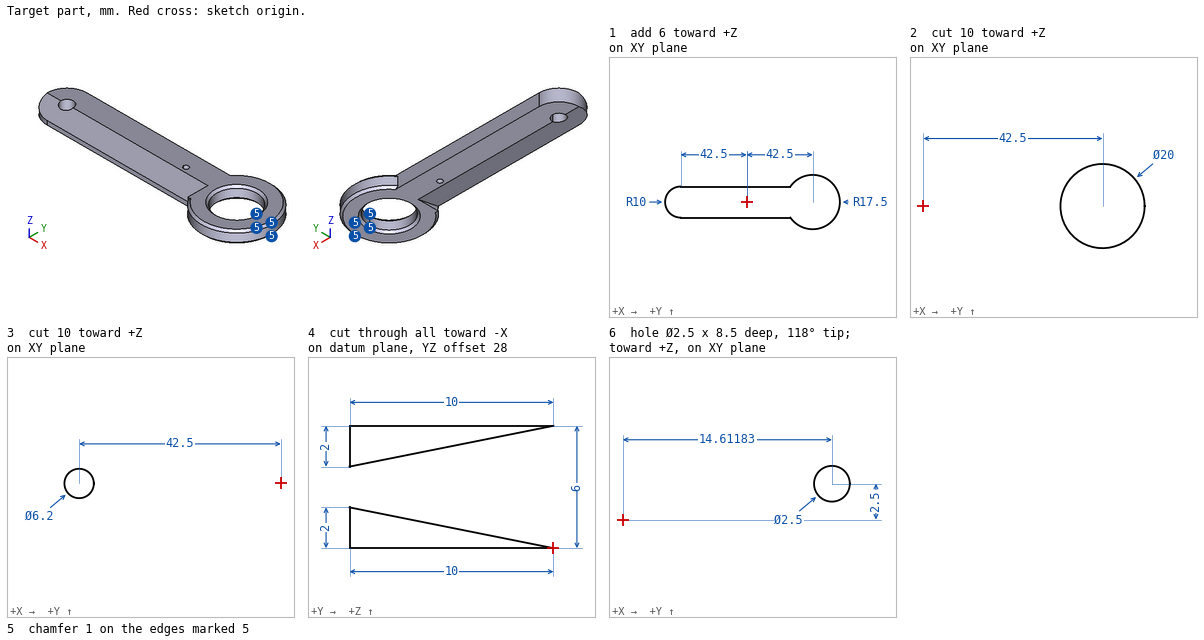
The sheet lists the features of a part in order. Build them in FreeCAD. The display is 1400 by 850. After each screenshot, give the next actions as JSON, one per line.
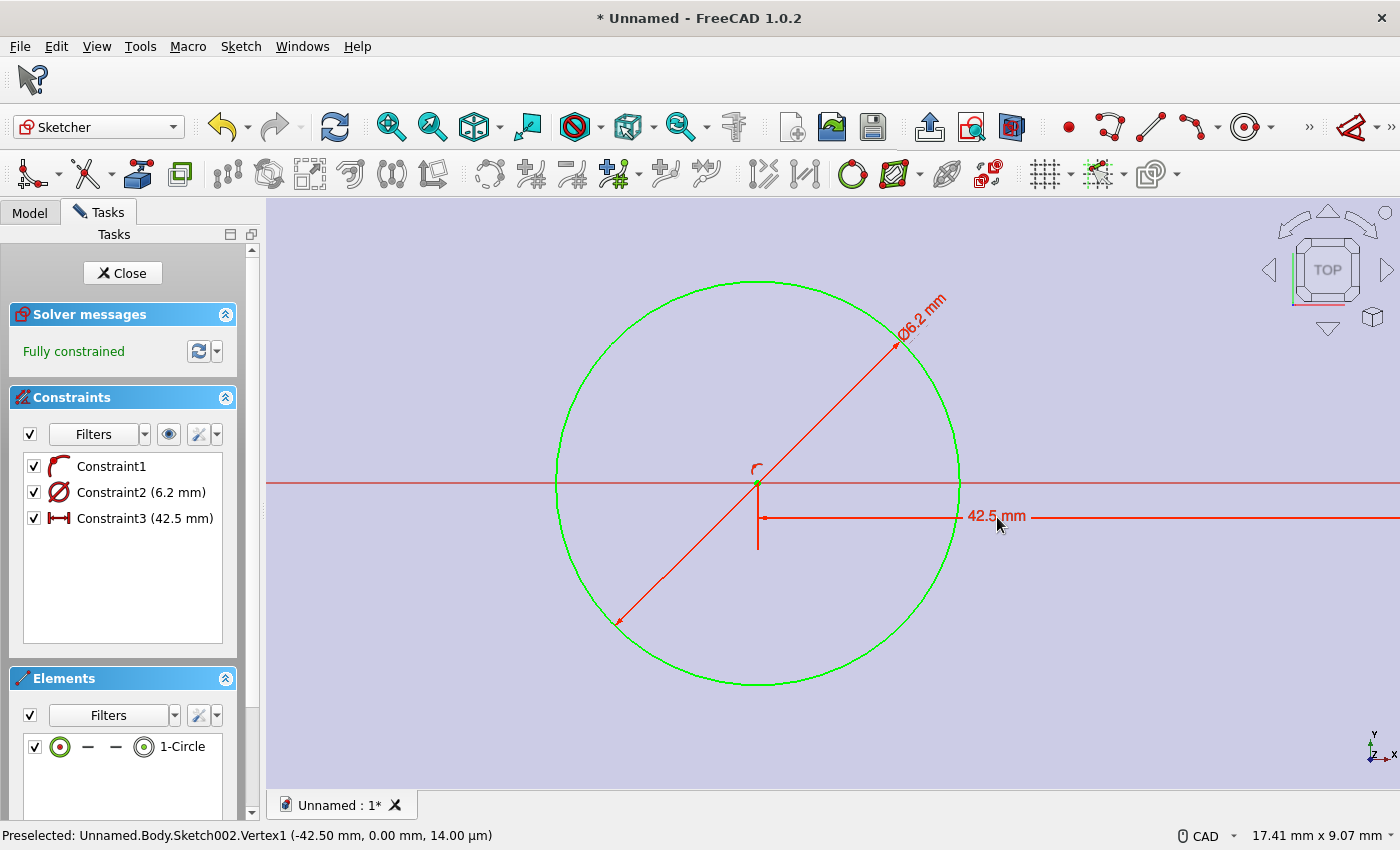
{"action": "left_click", "coordinate": [123, 273]}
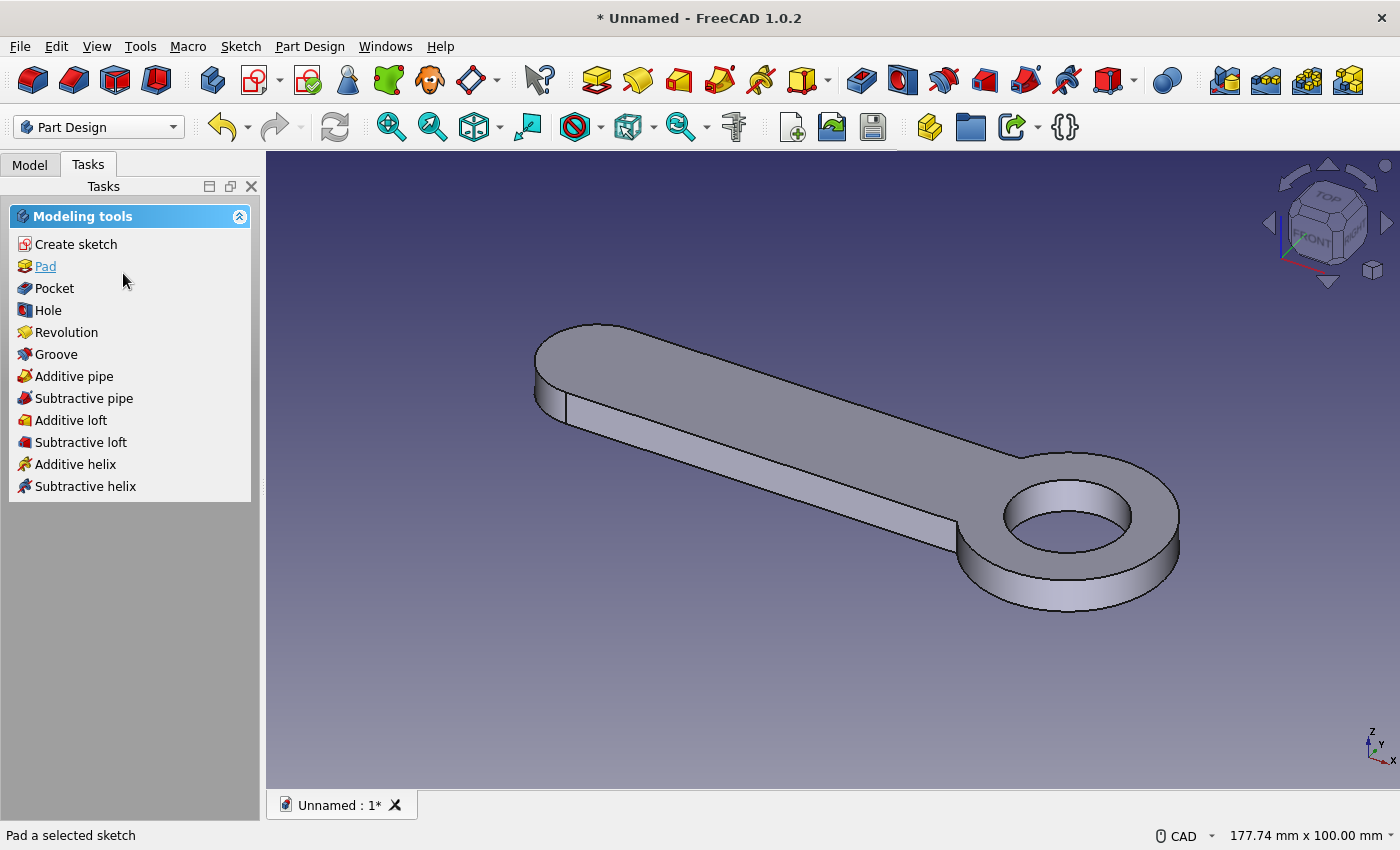
{"action": "left_click", "coordinate": [862, 80]}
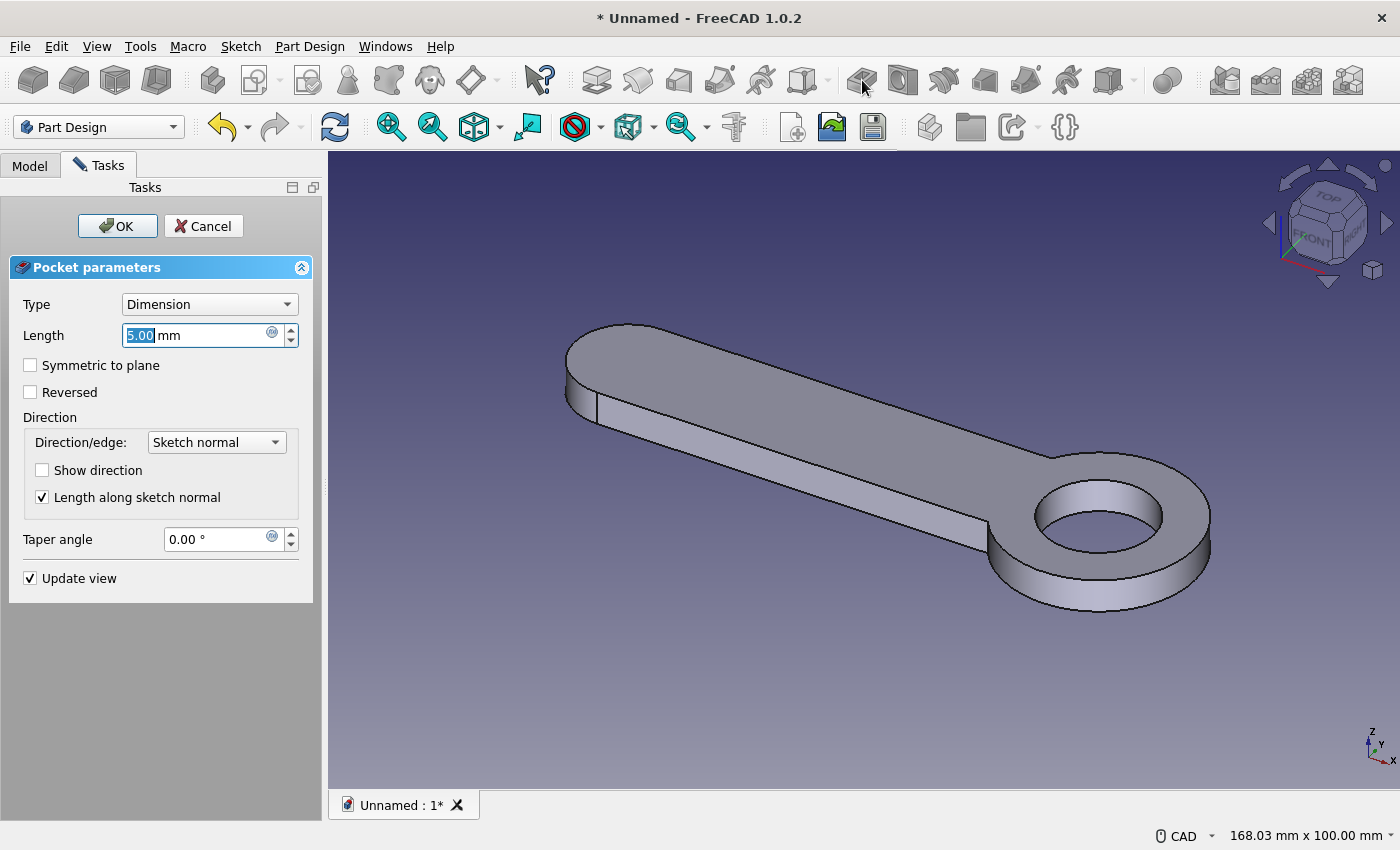
{"action": "type", "text": "10"}
{"action": "key", "text": "Tab"}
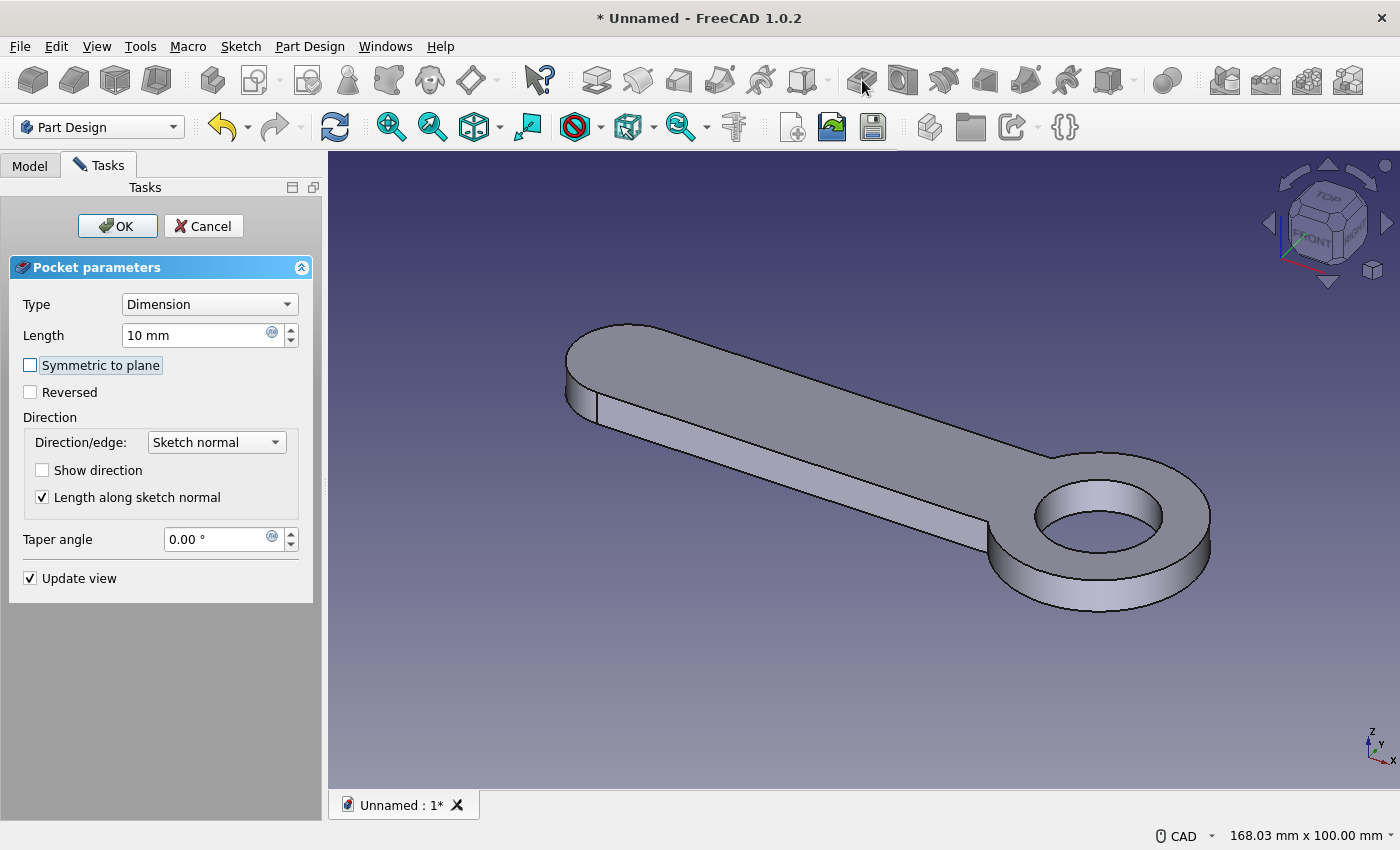
{"action": "left_click", "coordinate": [31, 392]}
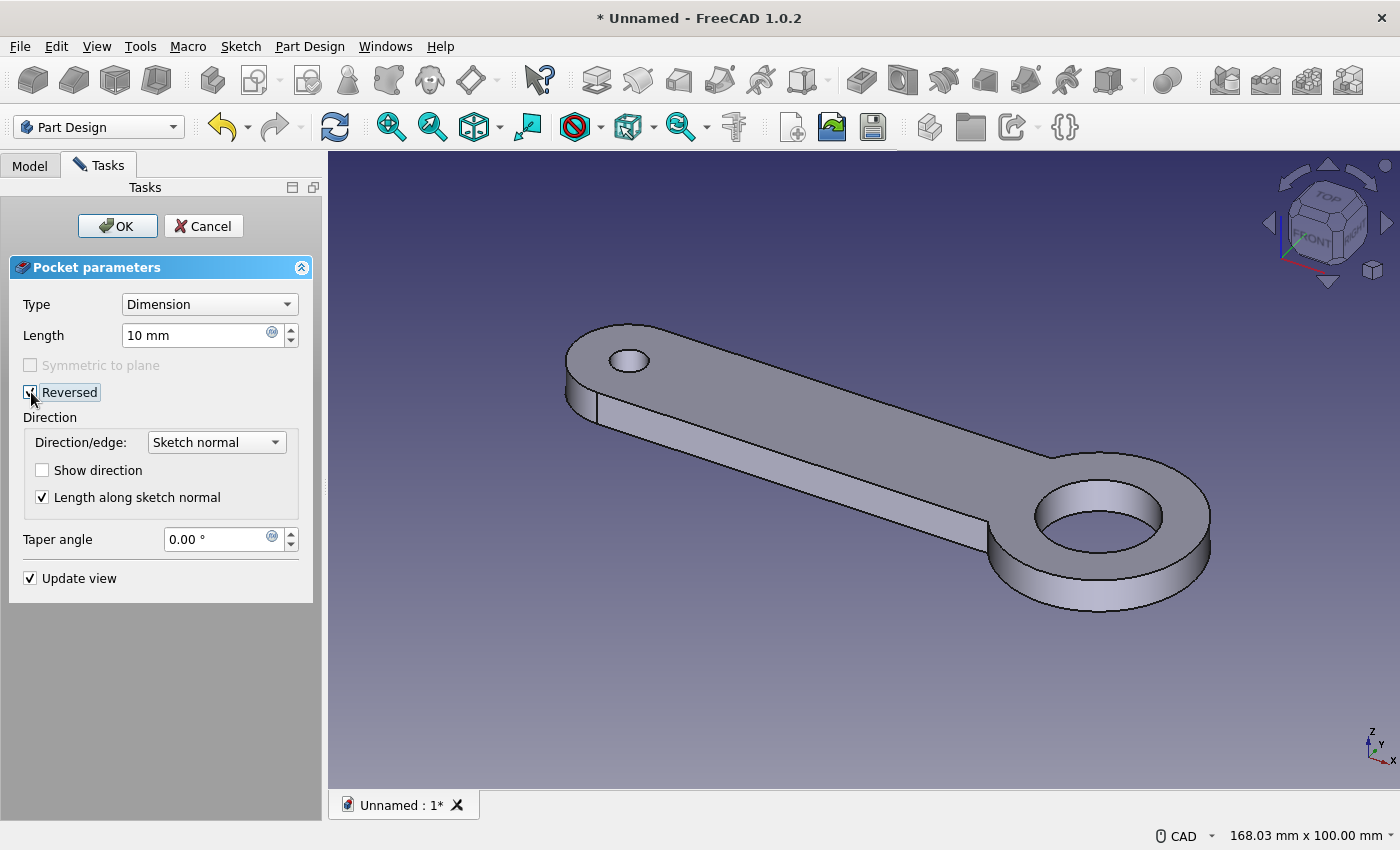
{"action": "left_click", "coordinate": [118, 226]}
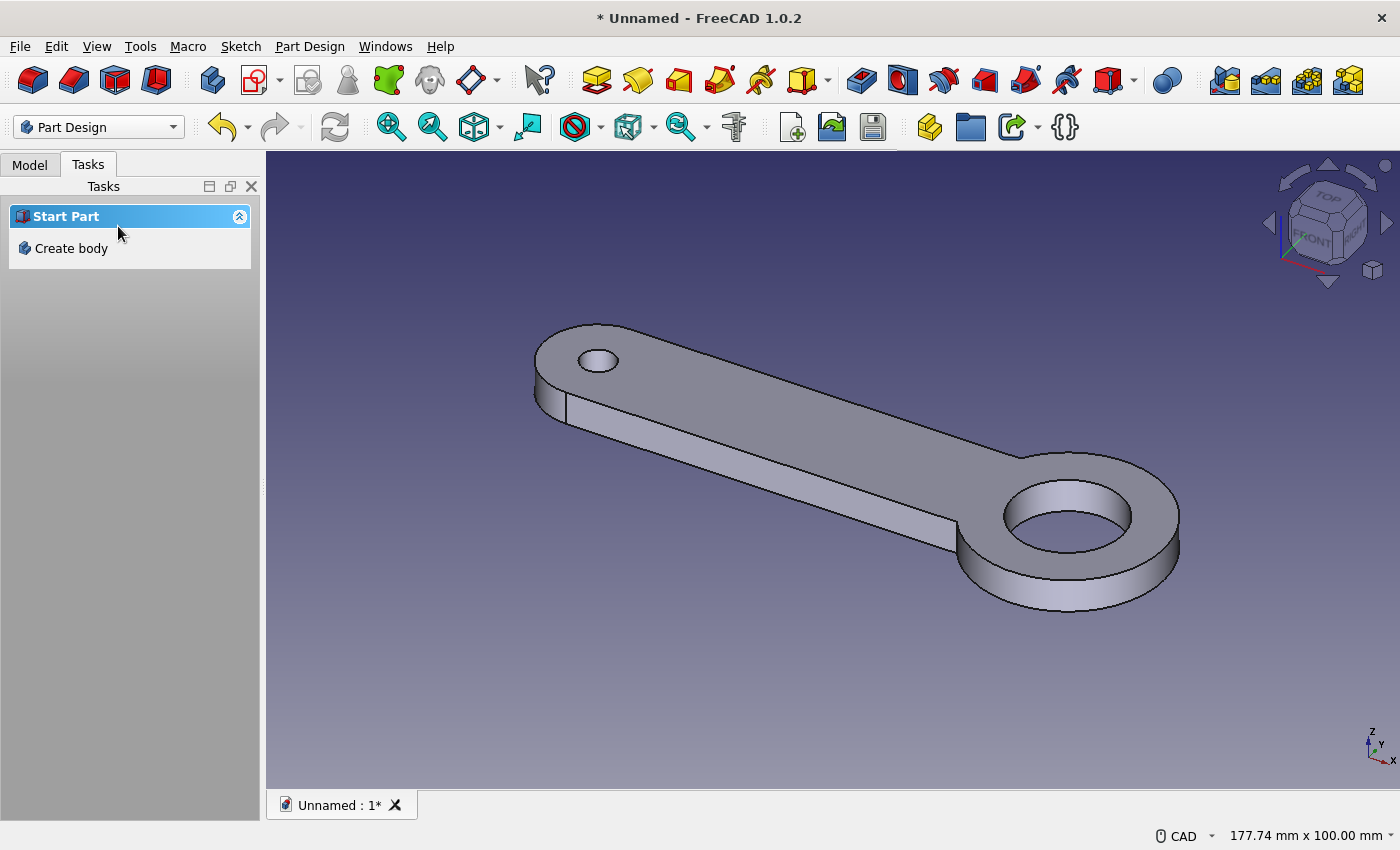
{"action": "left_click", "coordinate": [30, 164]}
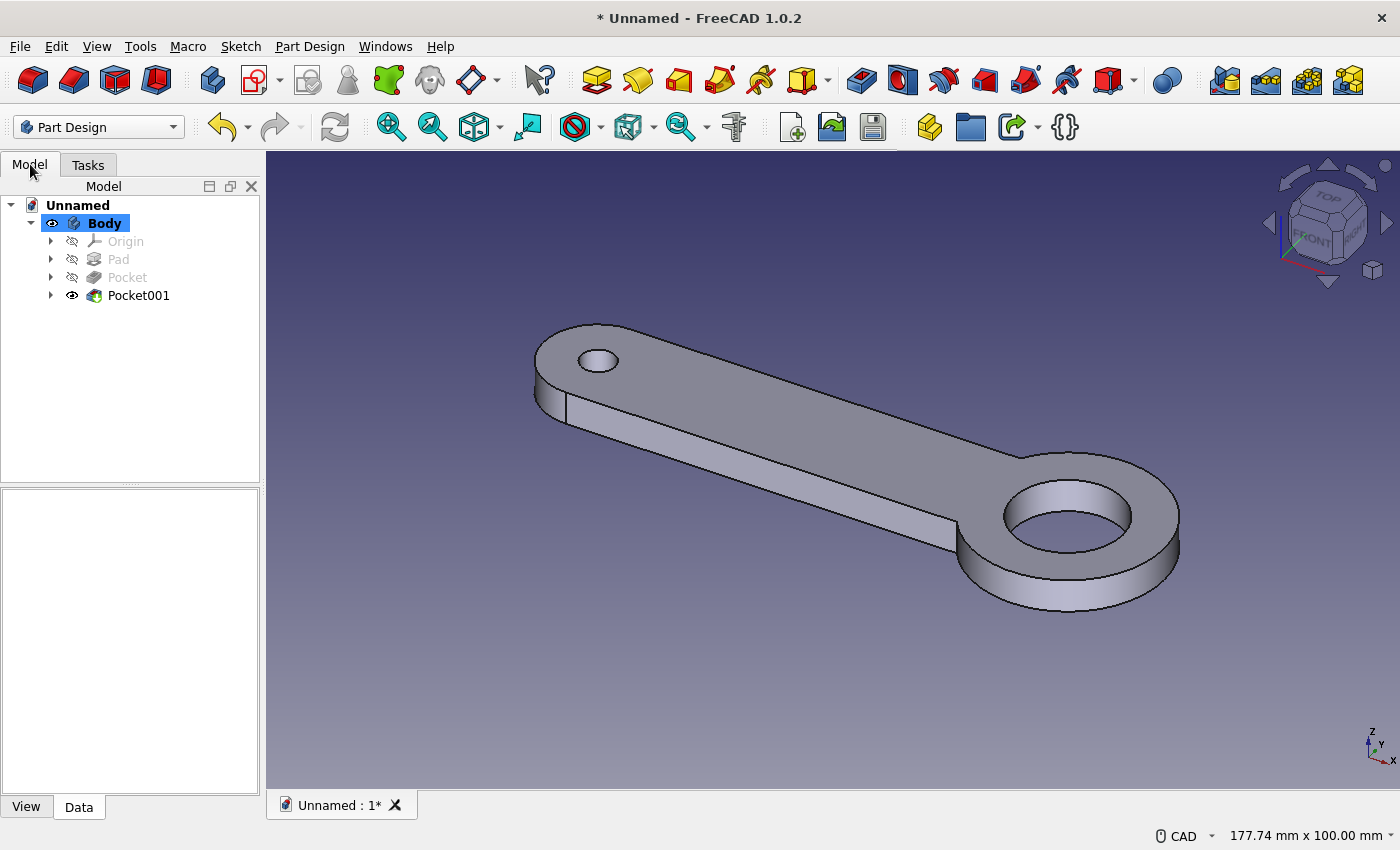
{"action": "left_click", "coordinate": [51, 241]}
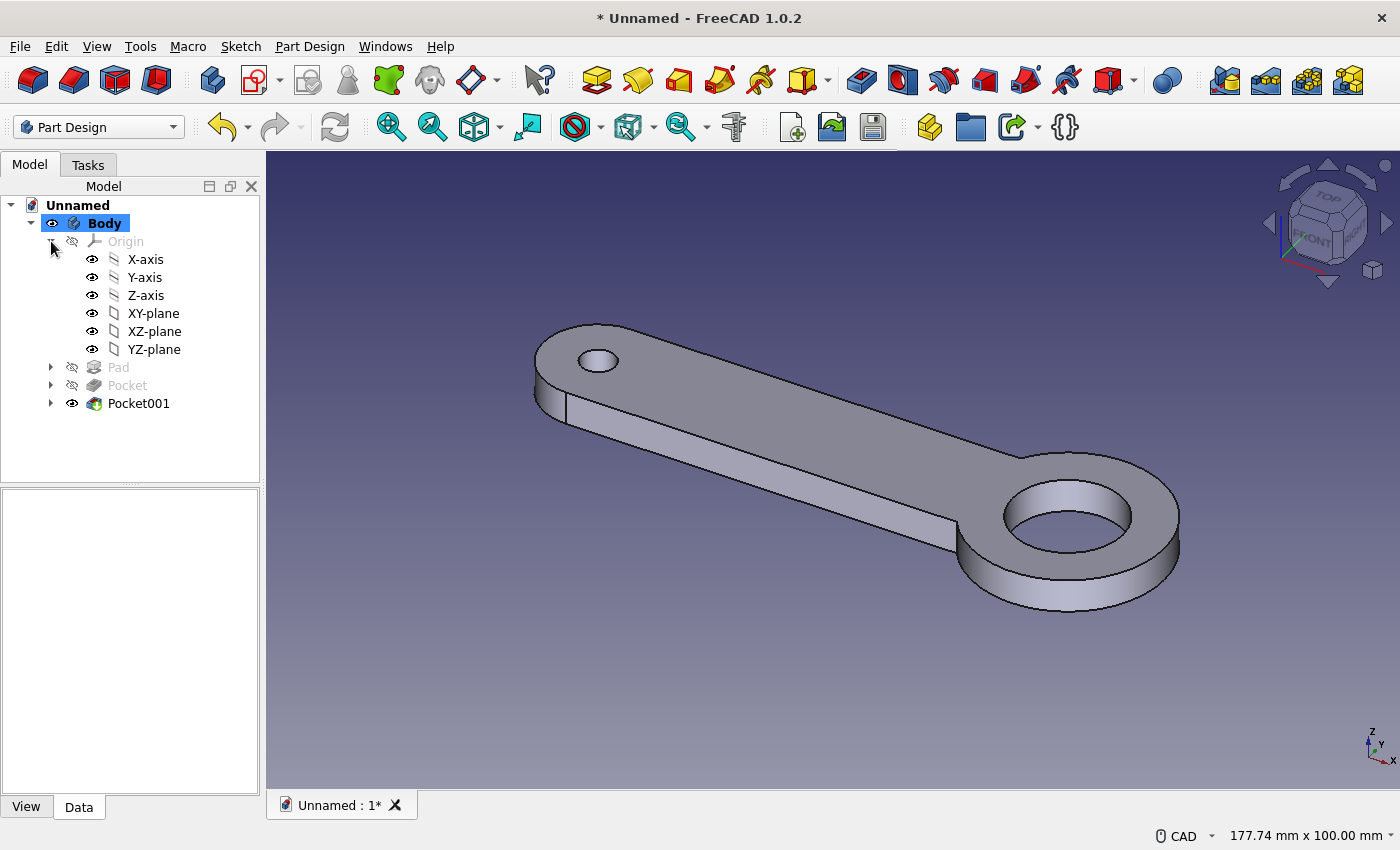
{"action": "left_click", "coordinate": [137, 349]}